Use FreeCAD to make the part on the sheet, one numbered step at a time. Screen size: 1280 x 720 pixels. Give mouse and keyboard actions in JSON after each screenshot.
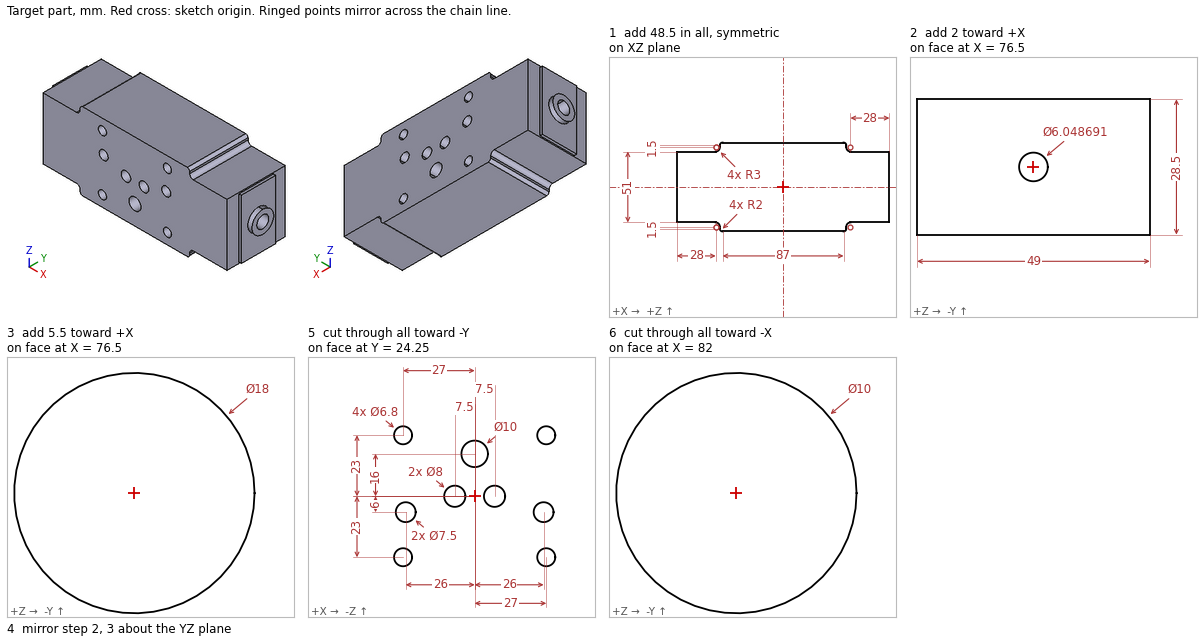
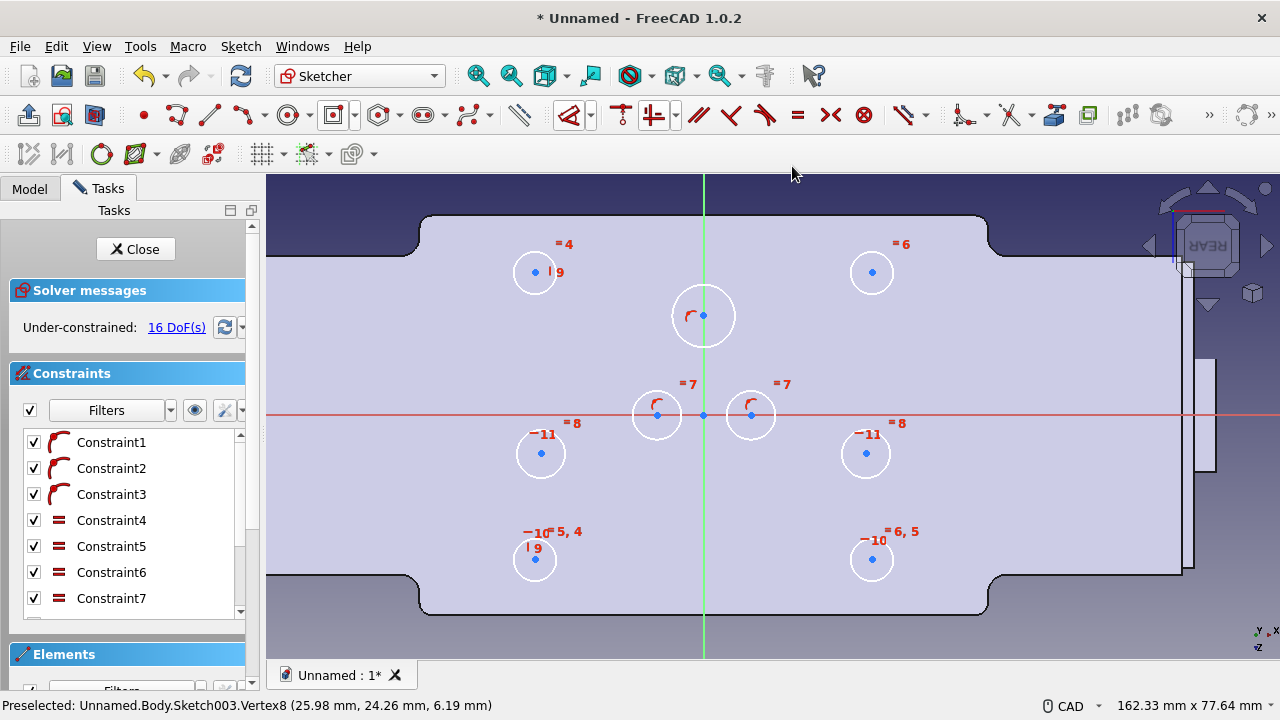
{"action": "left_click", "coordinate": [872, 560]}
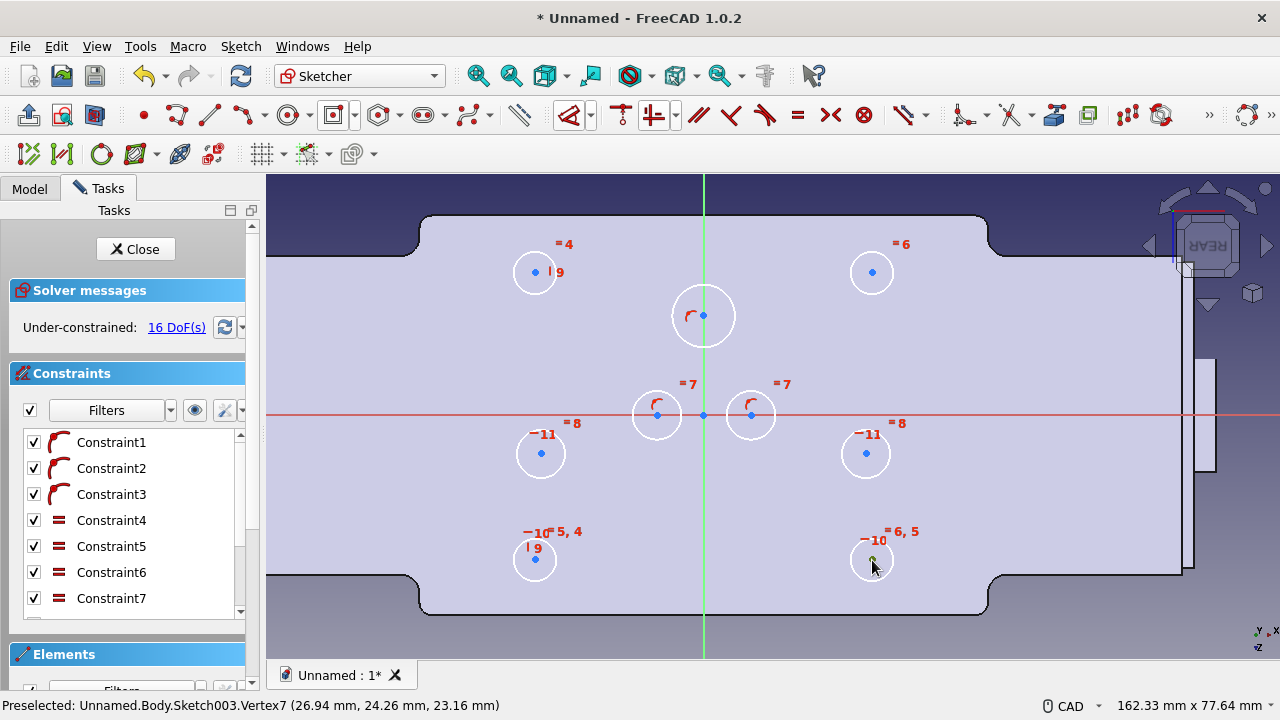
{"action": "left_click", "coordinate": [872, 273]}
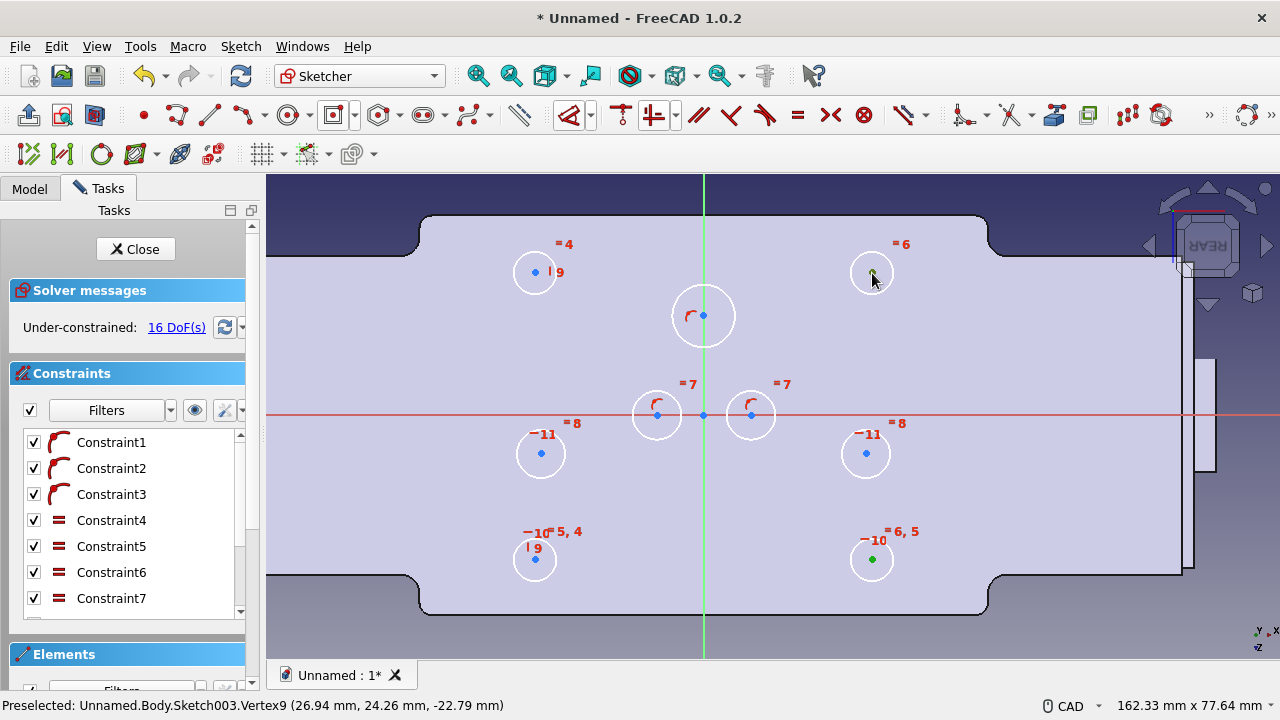
{"action": "key", "text": "v"}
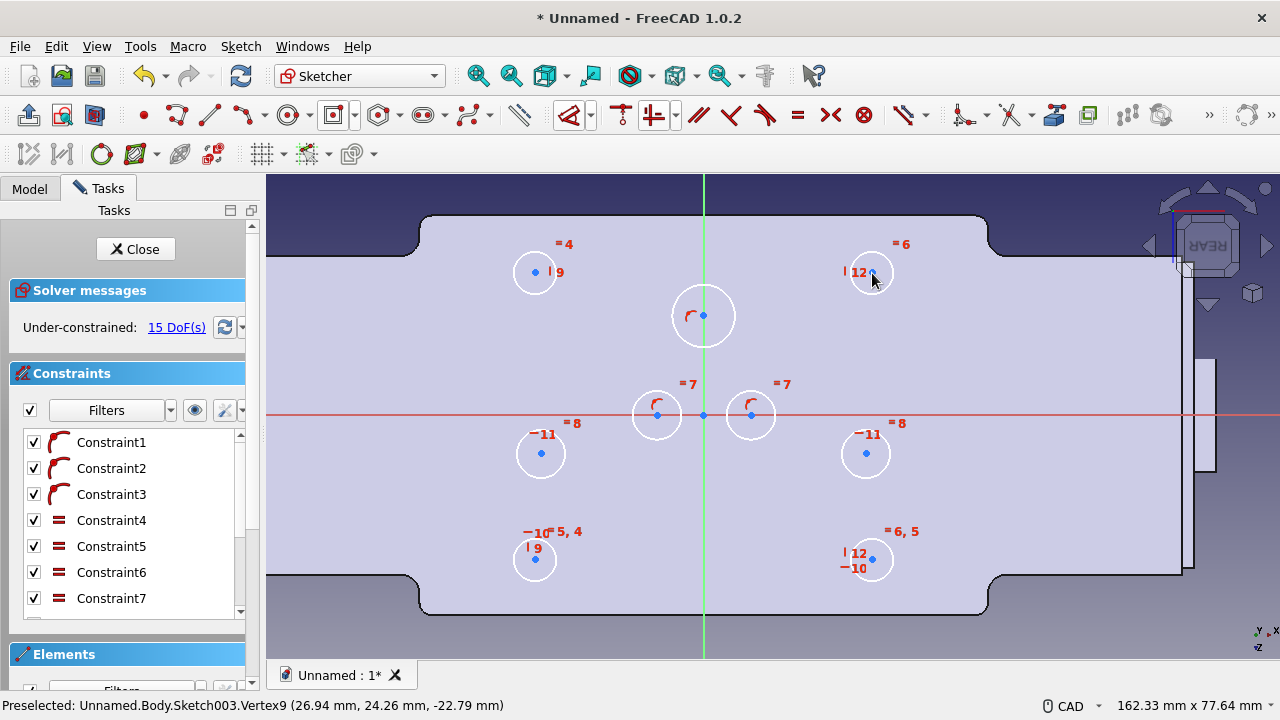
{"action": "left_click", "coordinate": [535, 273]}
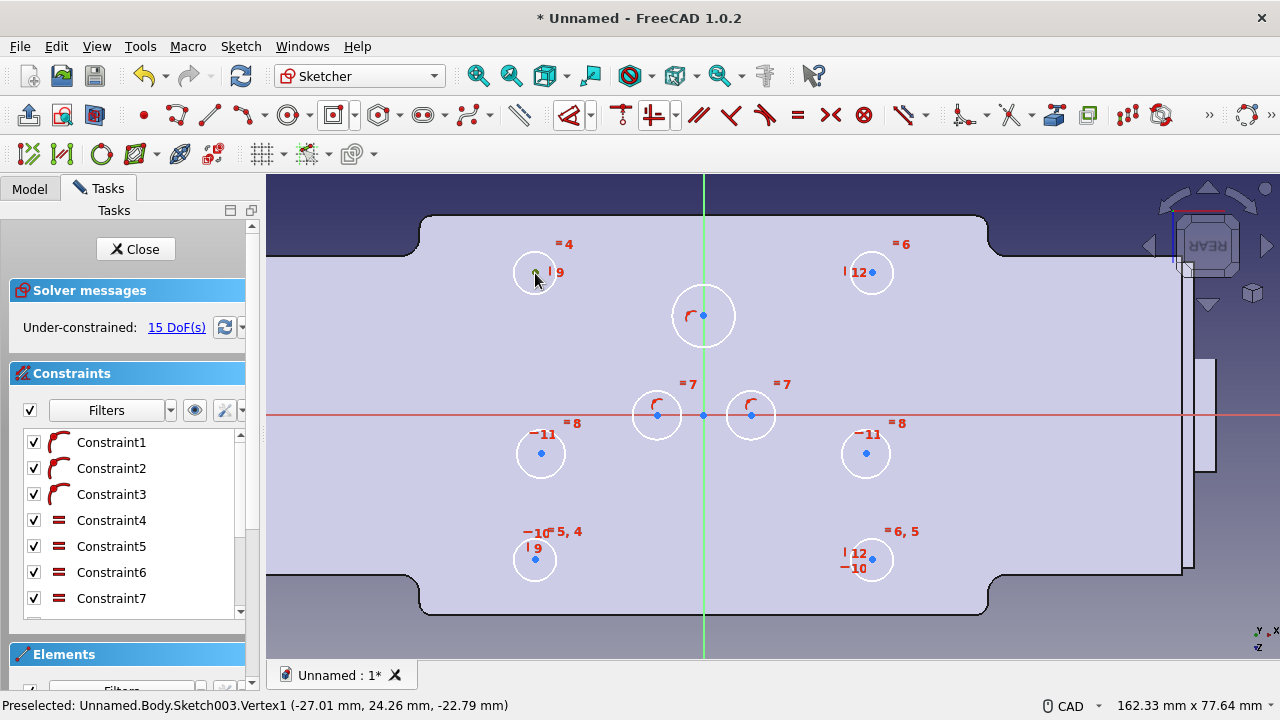
{"action": "left_click", "coordinate": [872, 273]}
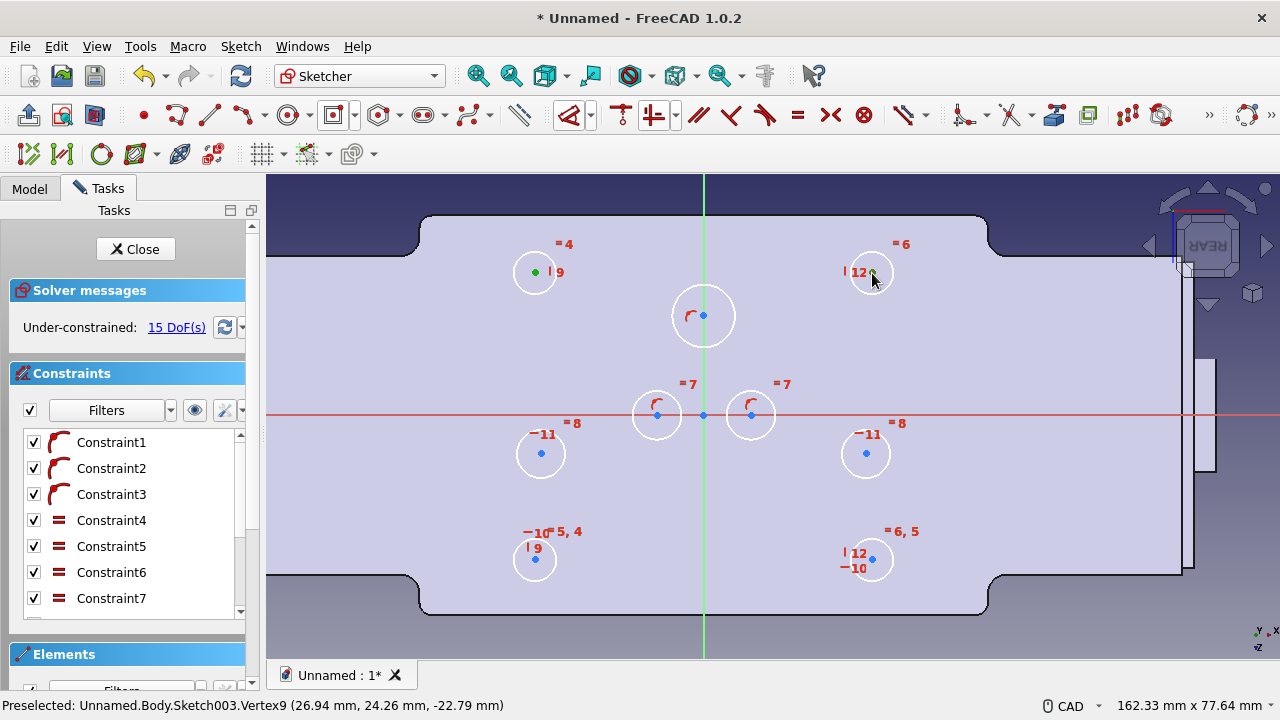
{"action": "left_click", "coordinate": [676, 116]}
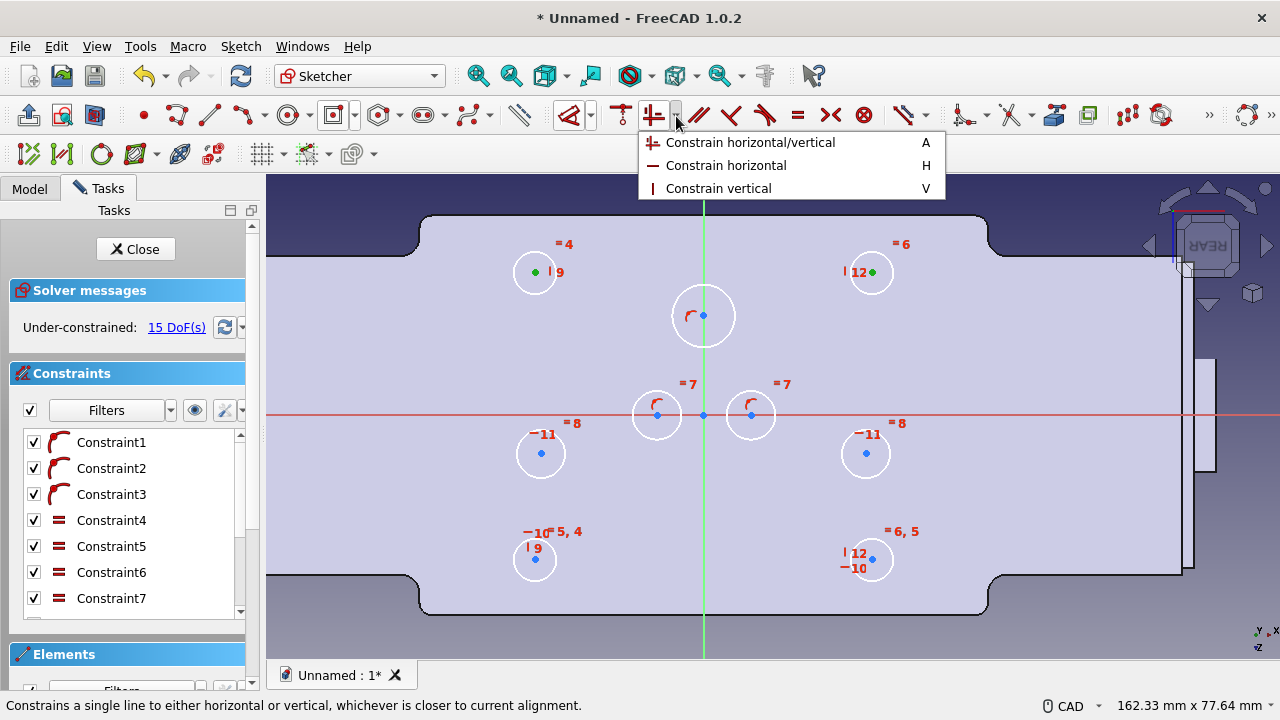
{"action": "left_click", "coordinate": [792, 166]}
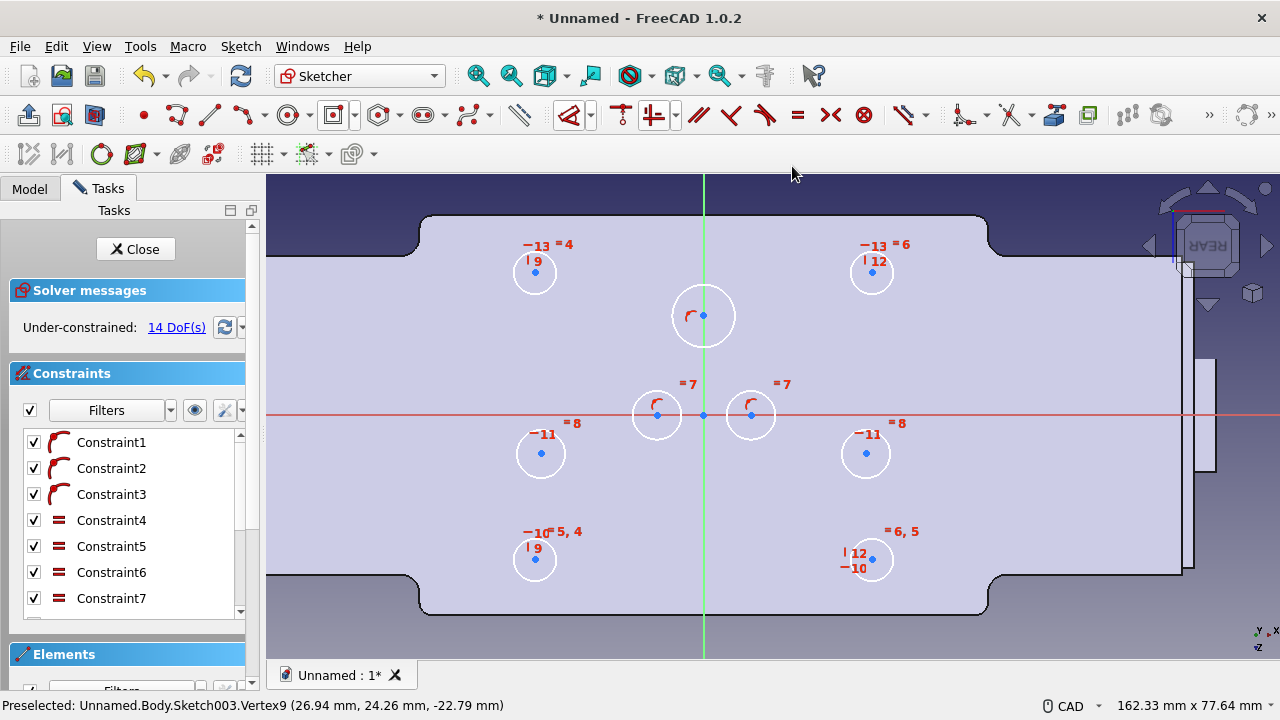
{"action": "left_click", "coordinate": [550, 258]}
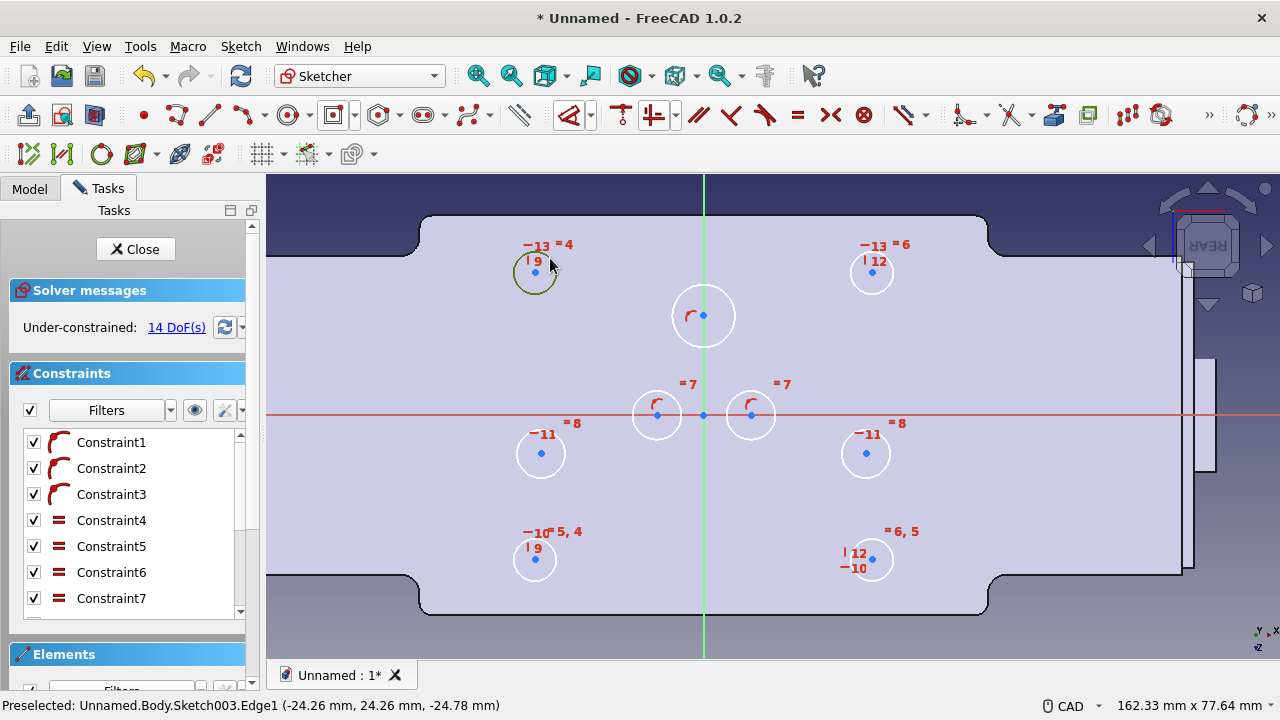
{"action": "left_click", "coordinate": [590, 116]}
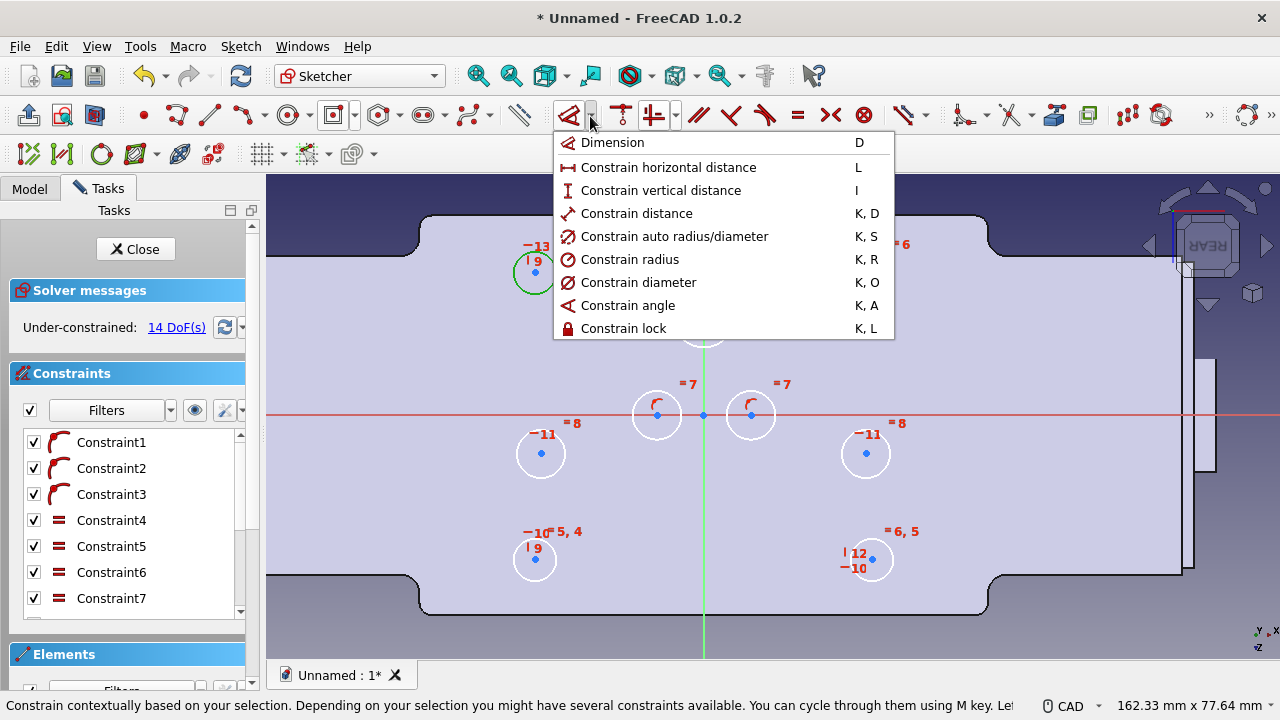
{"action": "left_click", "coordinate": [724, 282]}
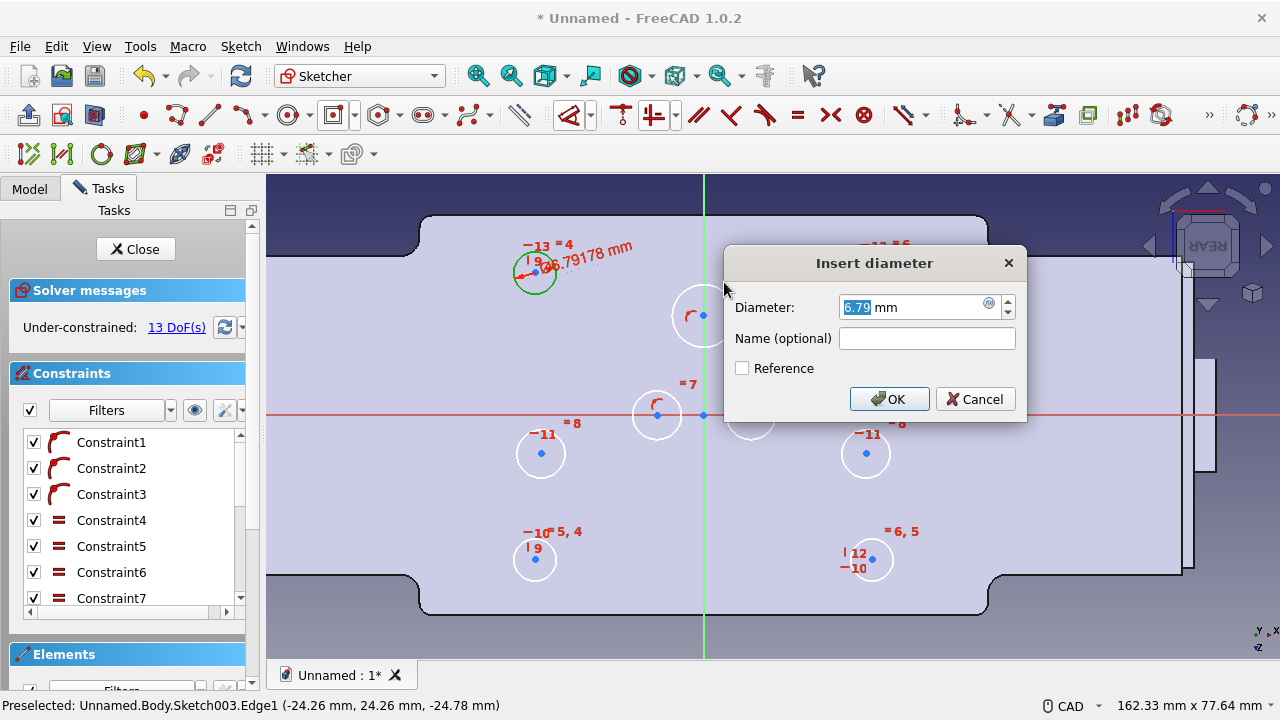
{"action": "type", "text": "6.8"}
{"action": "key", "text": "Return"}